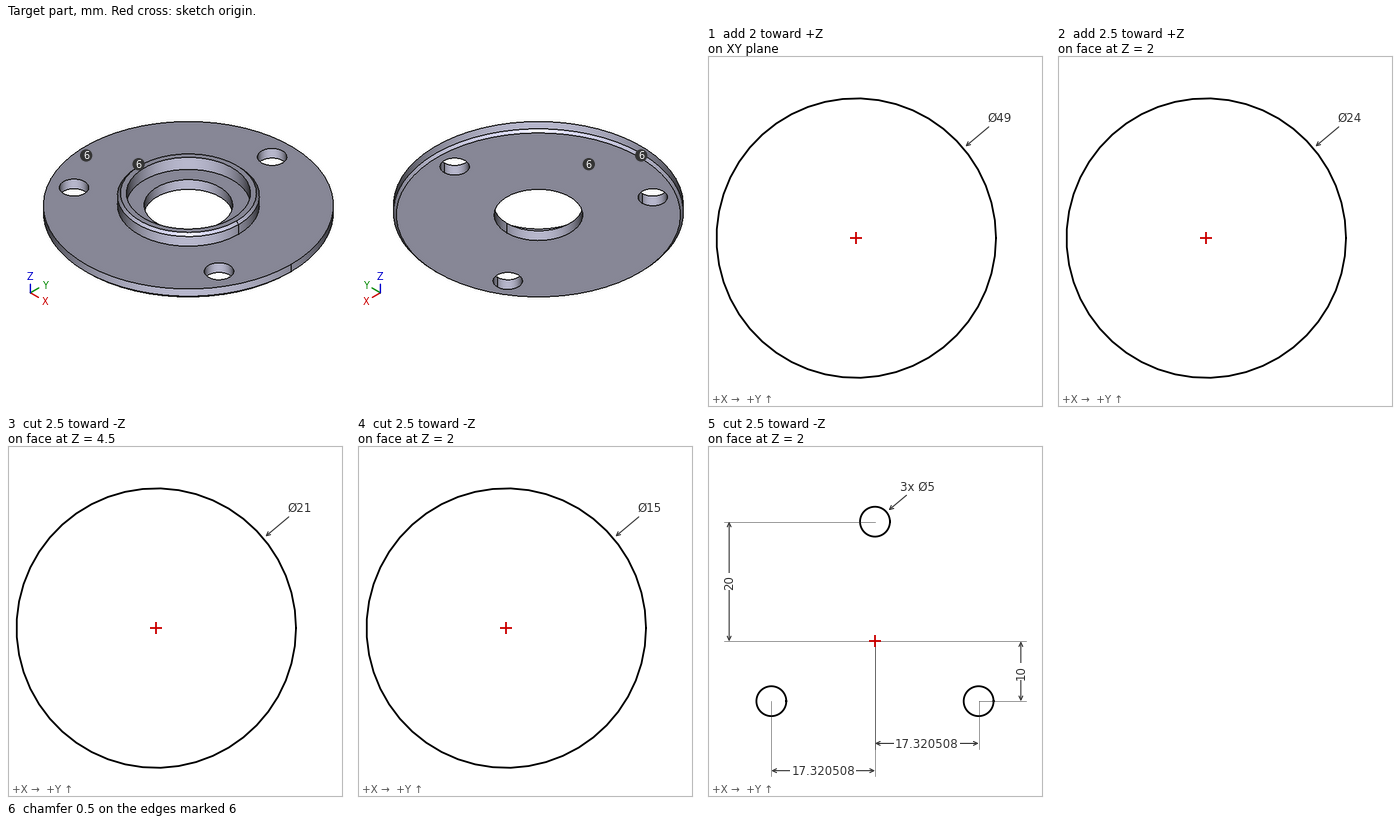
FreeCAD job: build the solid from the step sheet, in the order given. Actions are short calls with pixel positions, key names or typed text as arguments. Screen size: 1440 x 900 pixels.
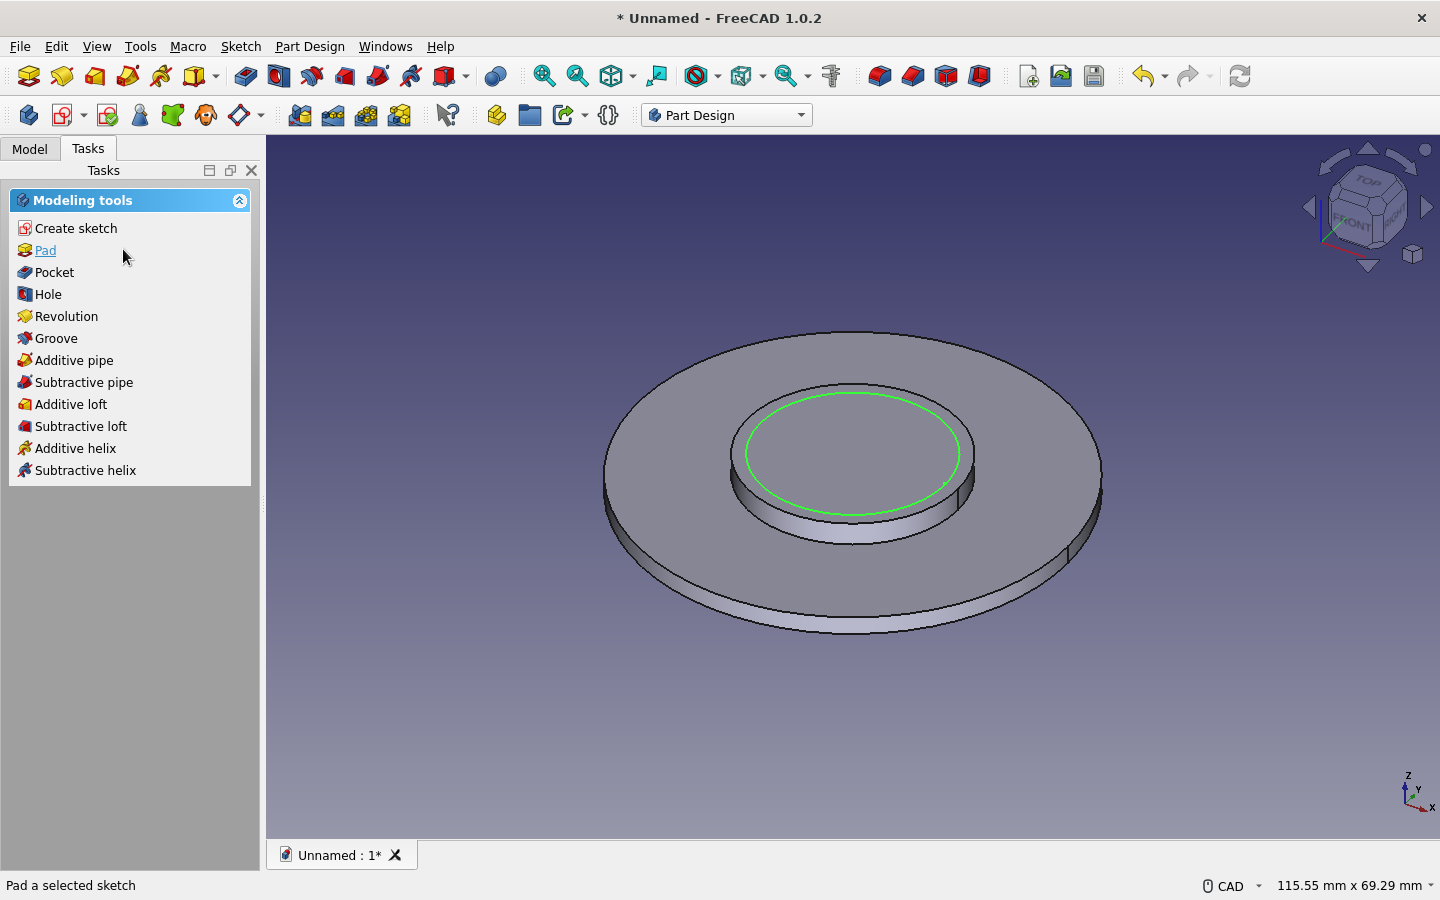
click(246, 76)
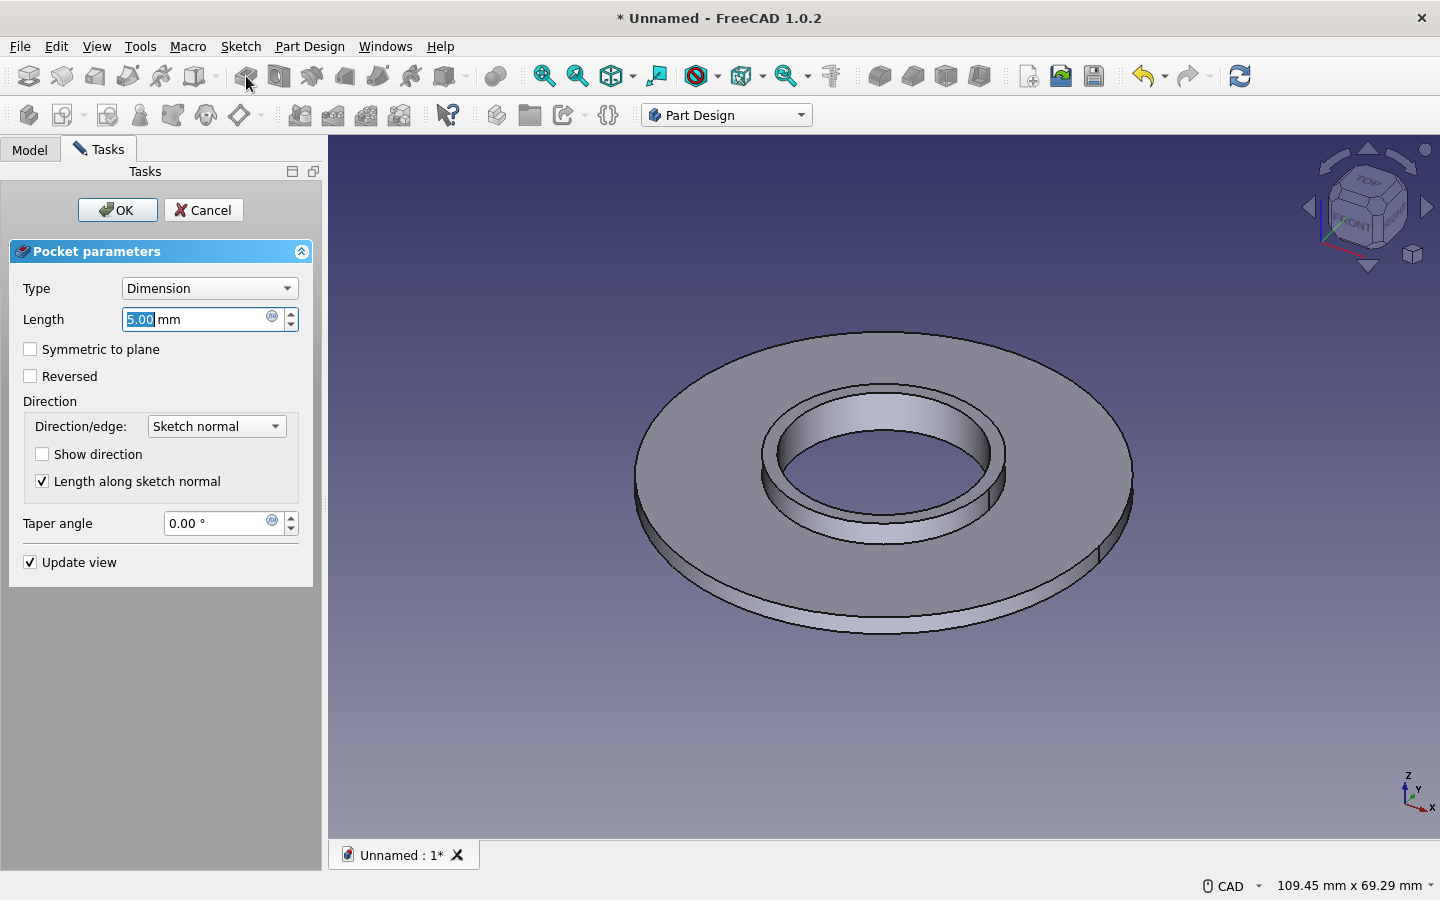
text(2.5)
key(Tab)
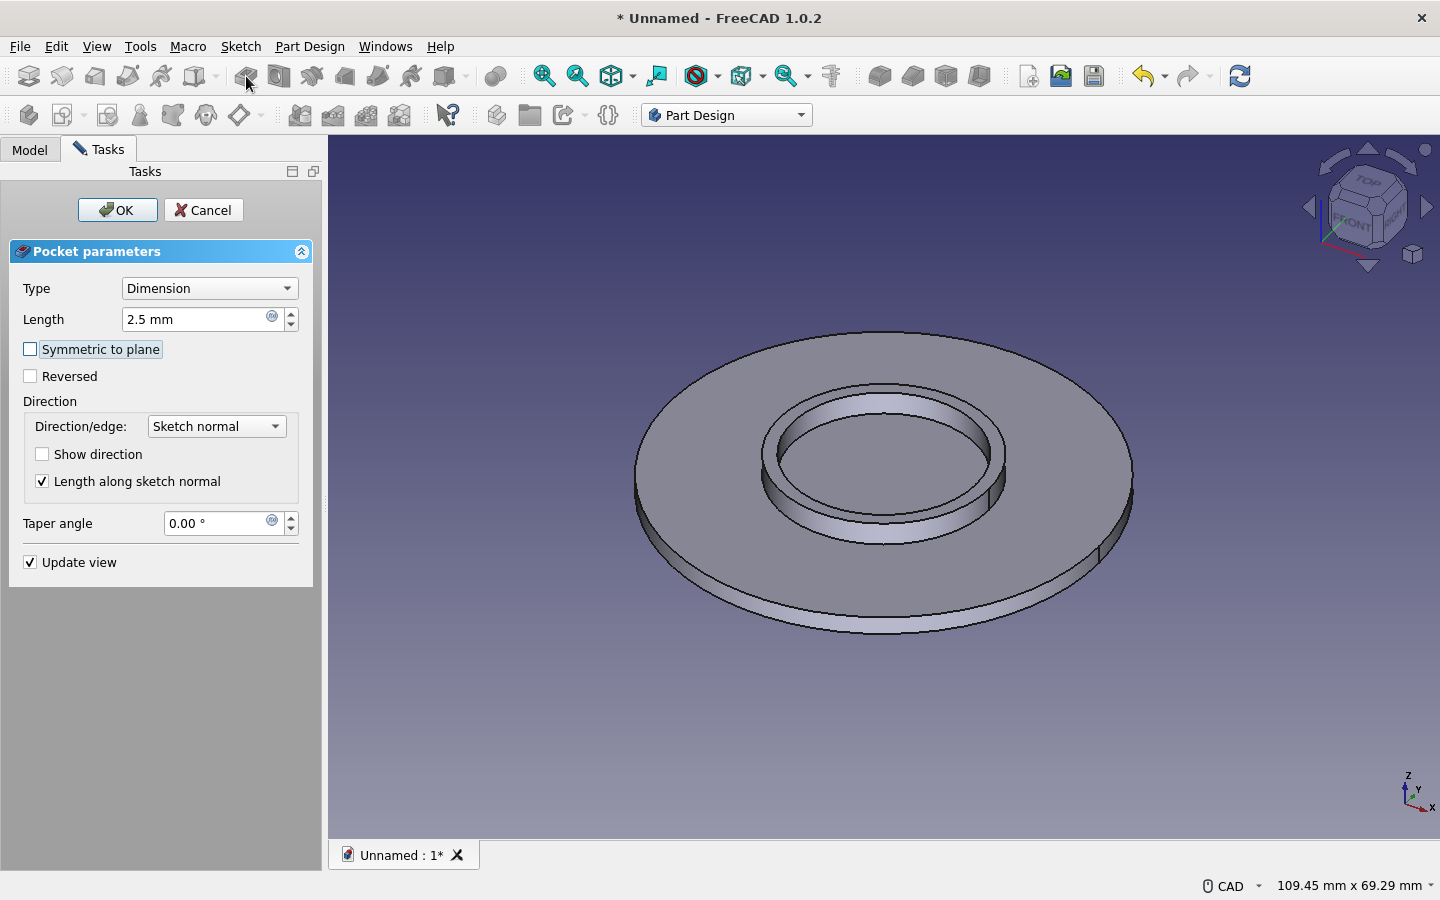
click(118, 210)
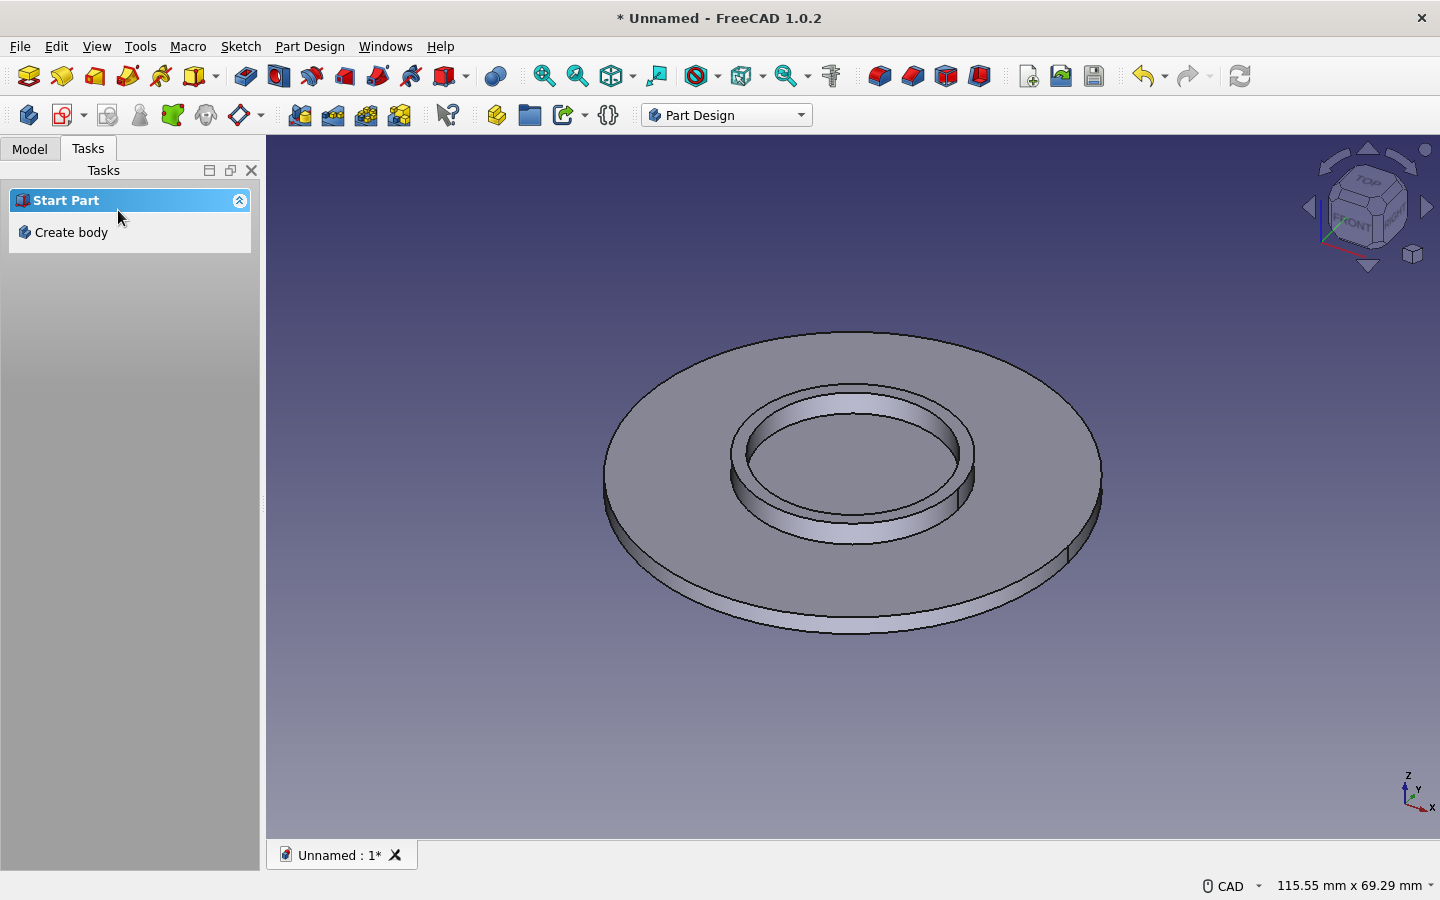
click(1047, 444)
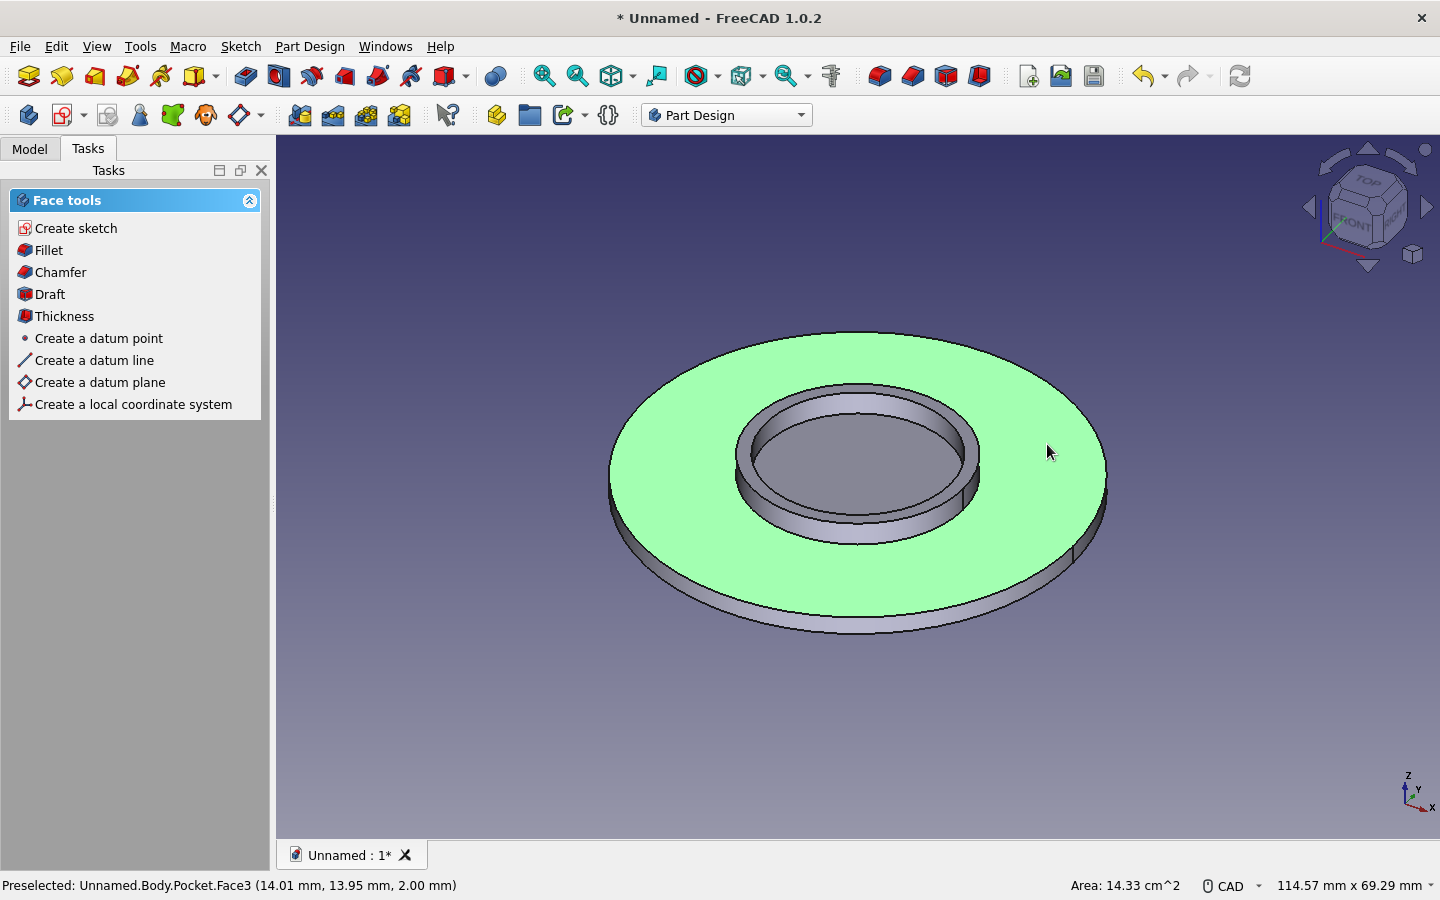
click(62, 116)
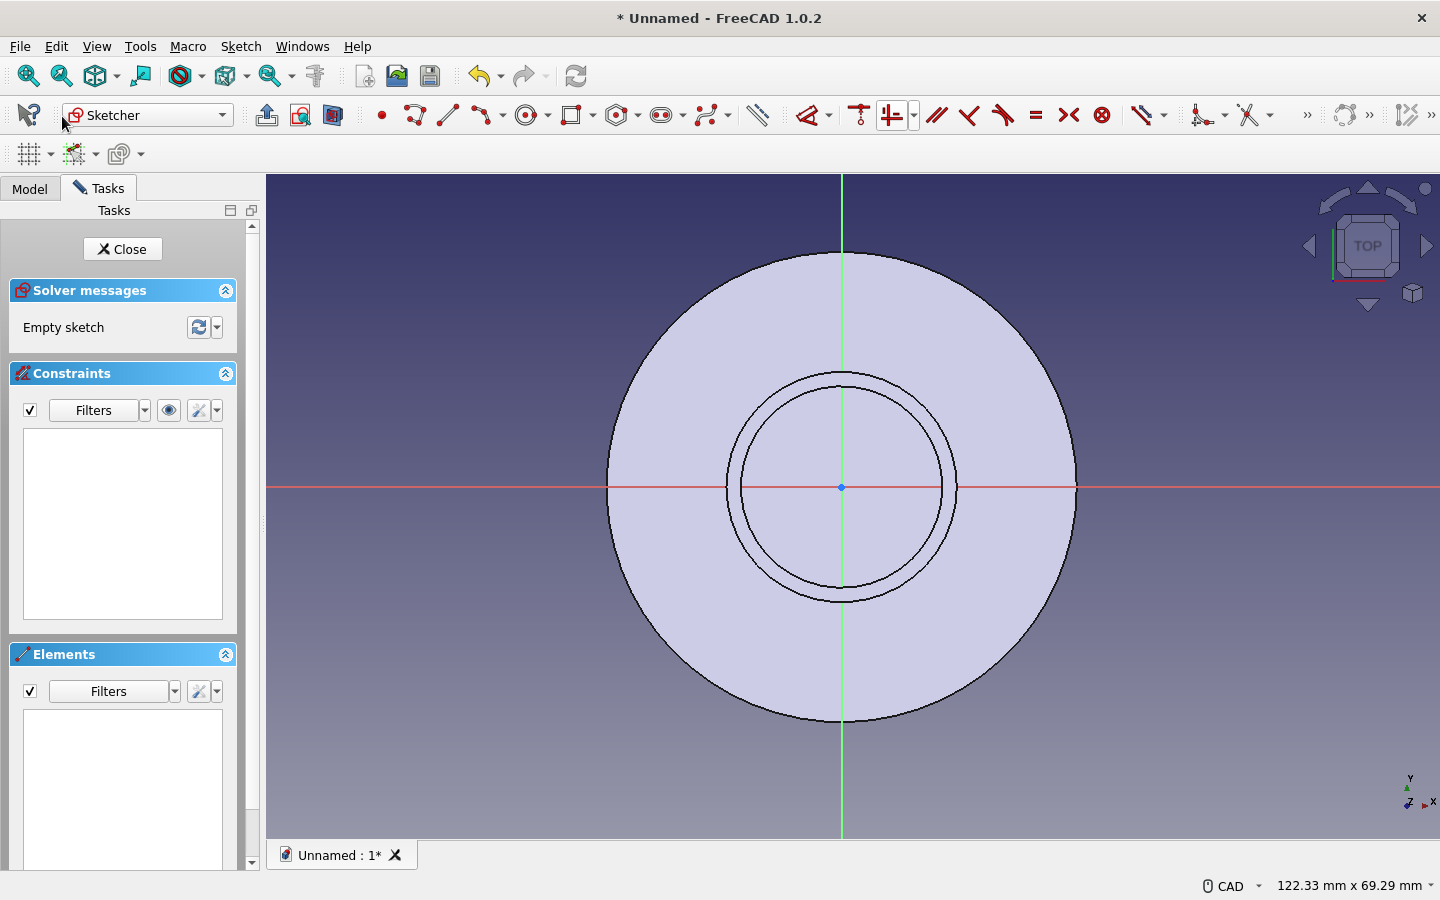
scroll(875, 476, up, 5)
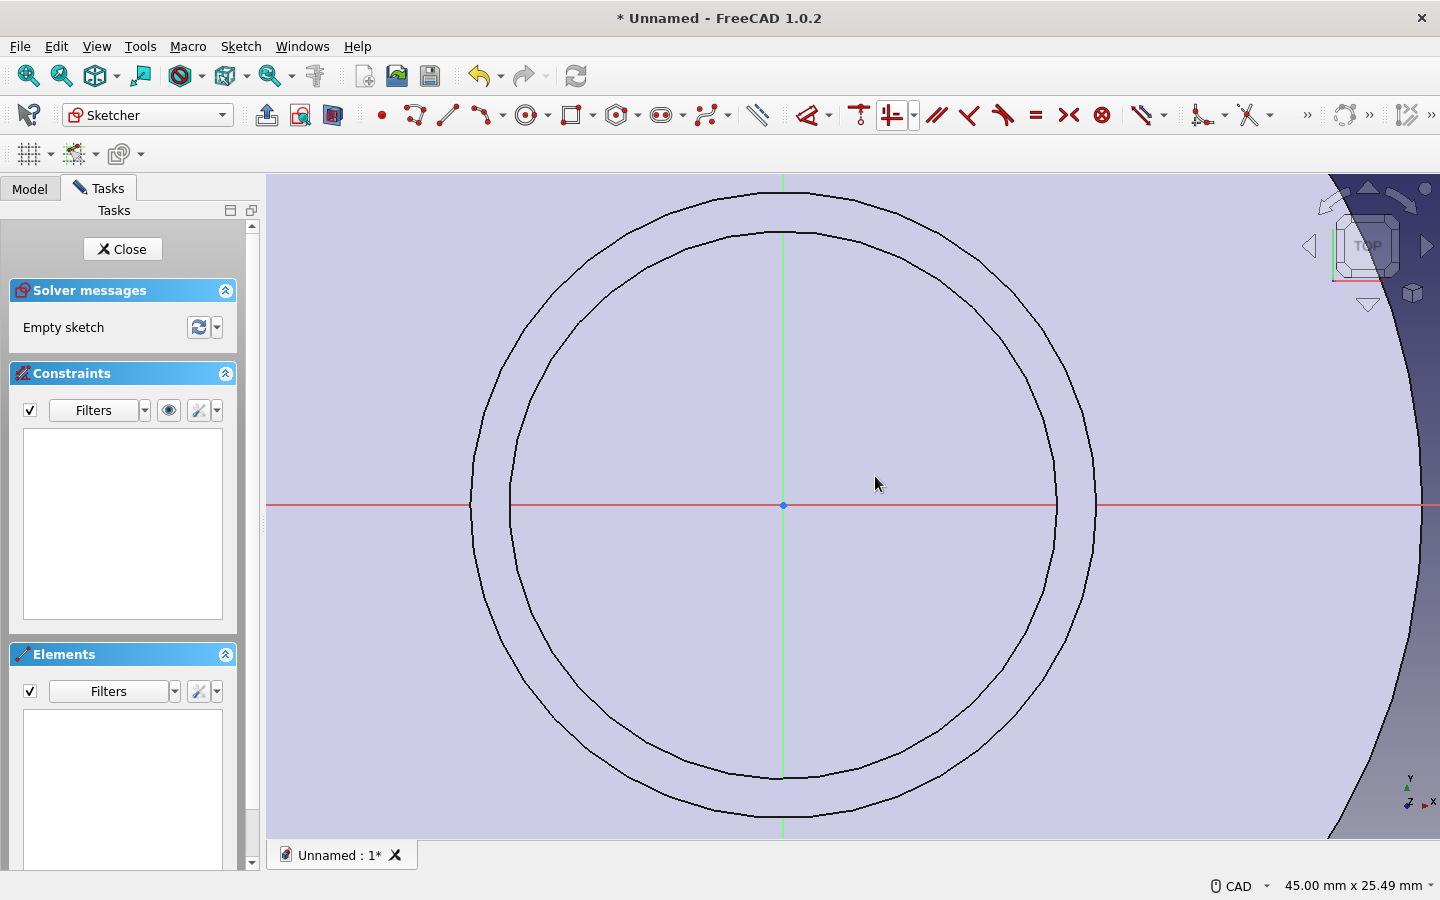
click(526, 116)